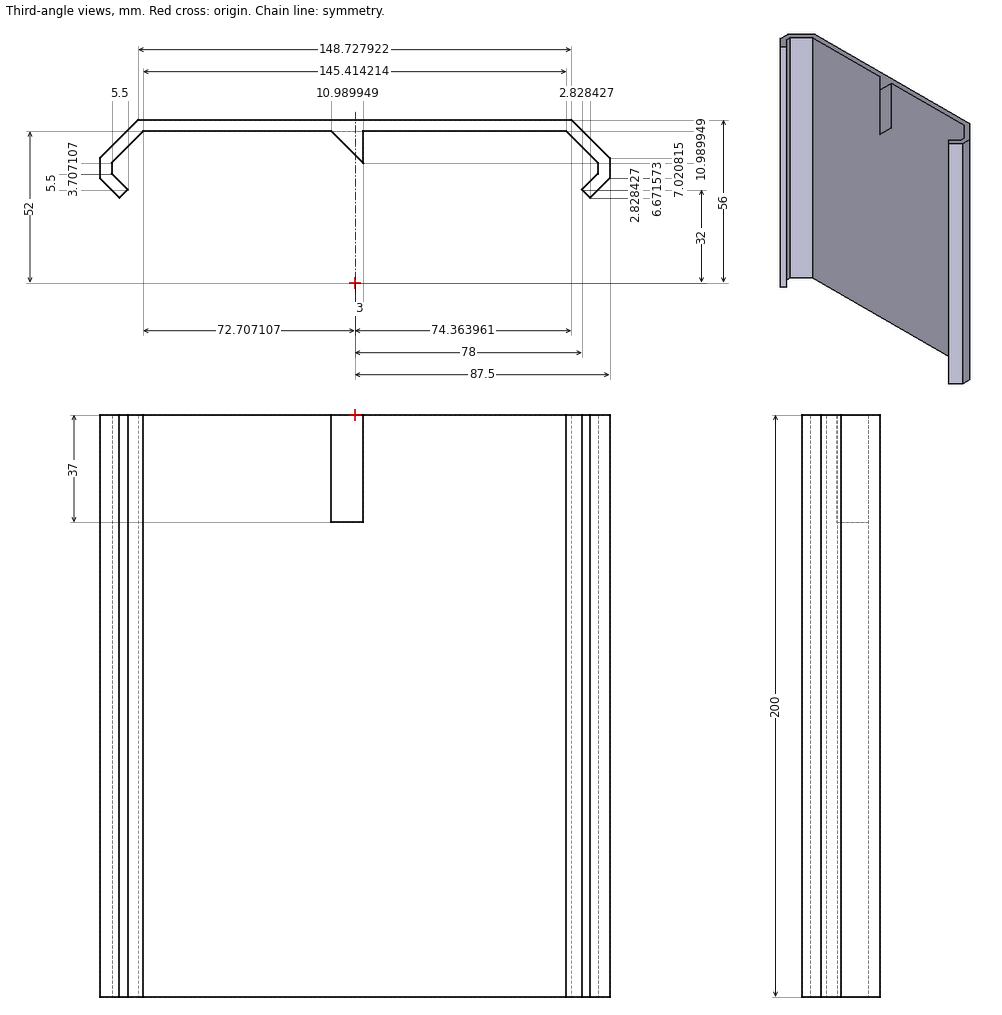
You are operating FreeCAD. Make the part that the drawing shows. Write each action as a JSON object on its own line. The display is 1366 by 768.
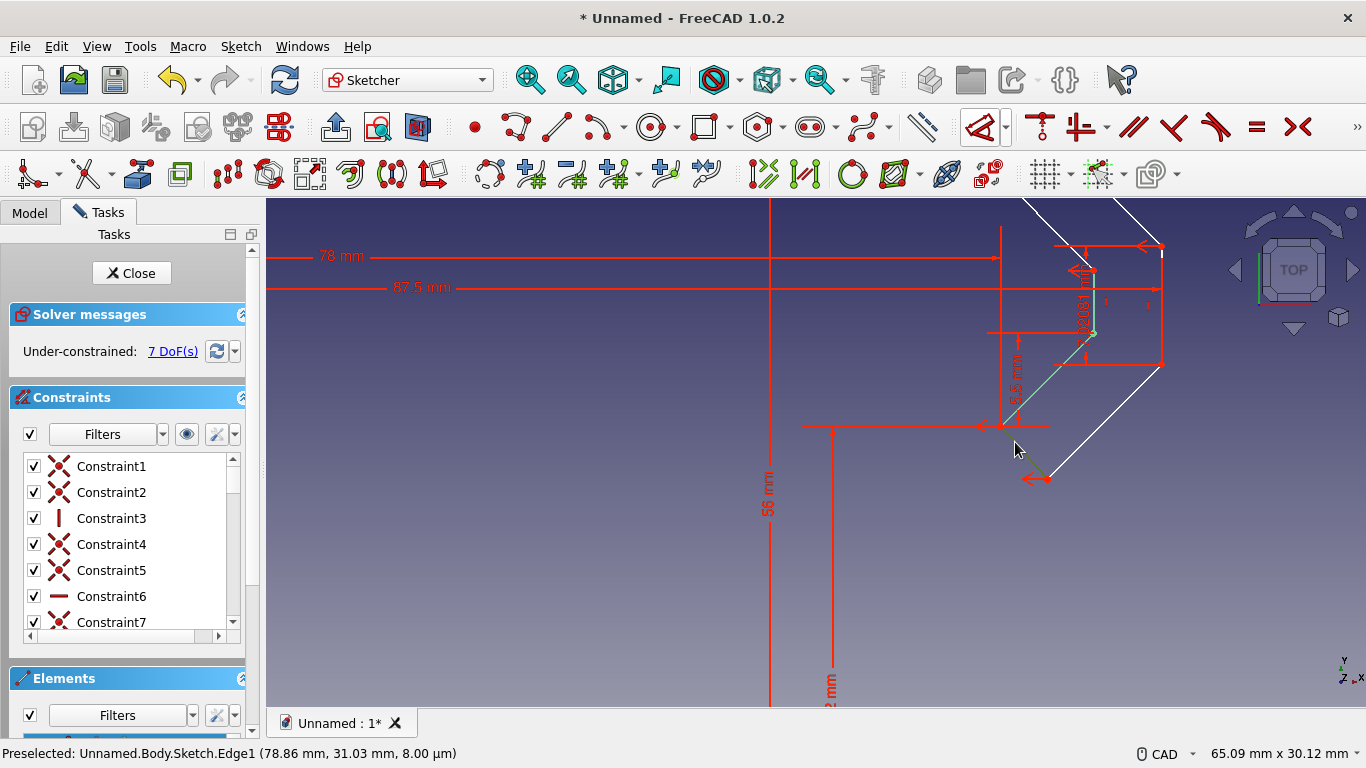
{"action": "left_click", "coordinate": [1006, 128]}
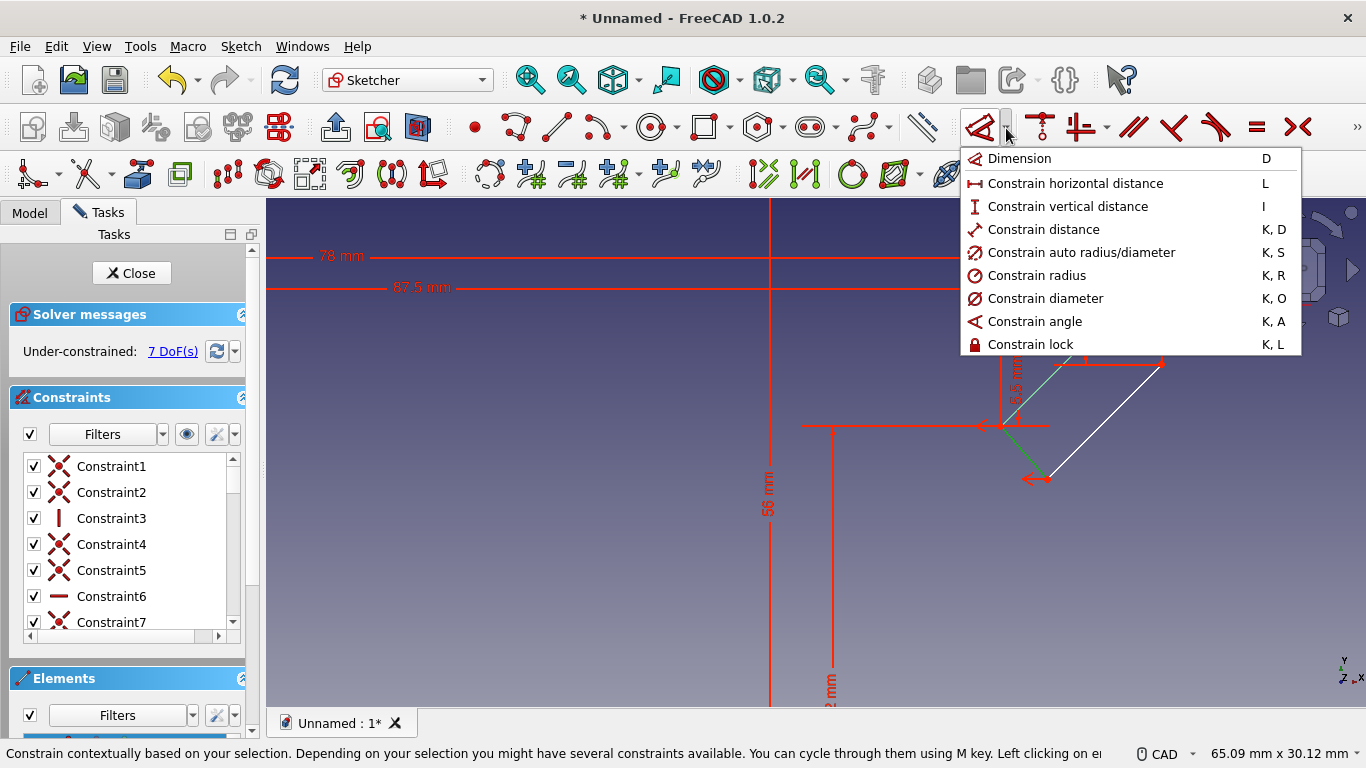
{"action": "left_click", "coordinate": [1131, 184]}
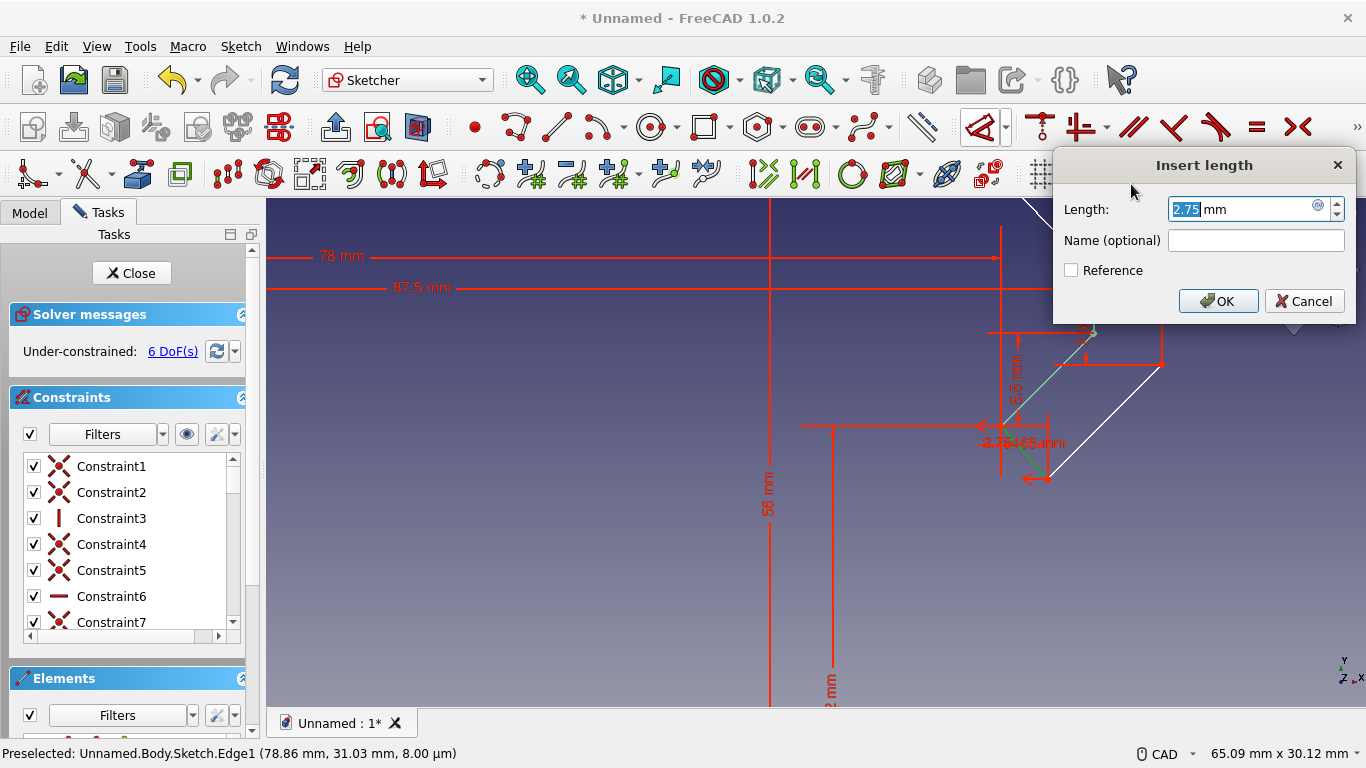
{"action": "type", "text": "2.828427"}
{"action": "key", "text": "Return"}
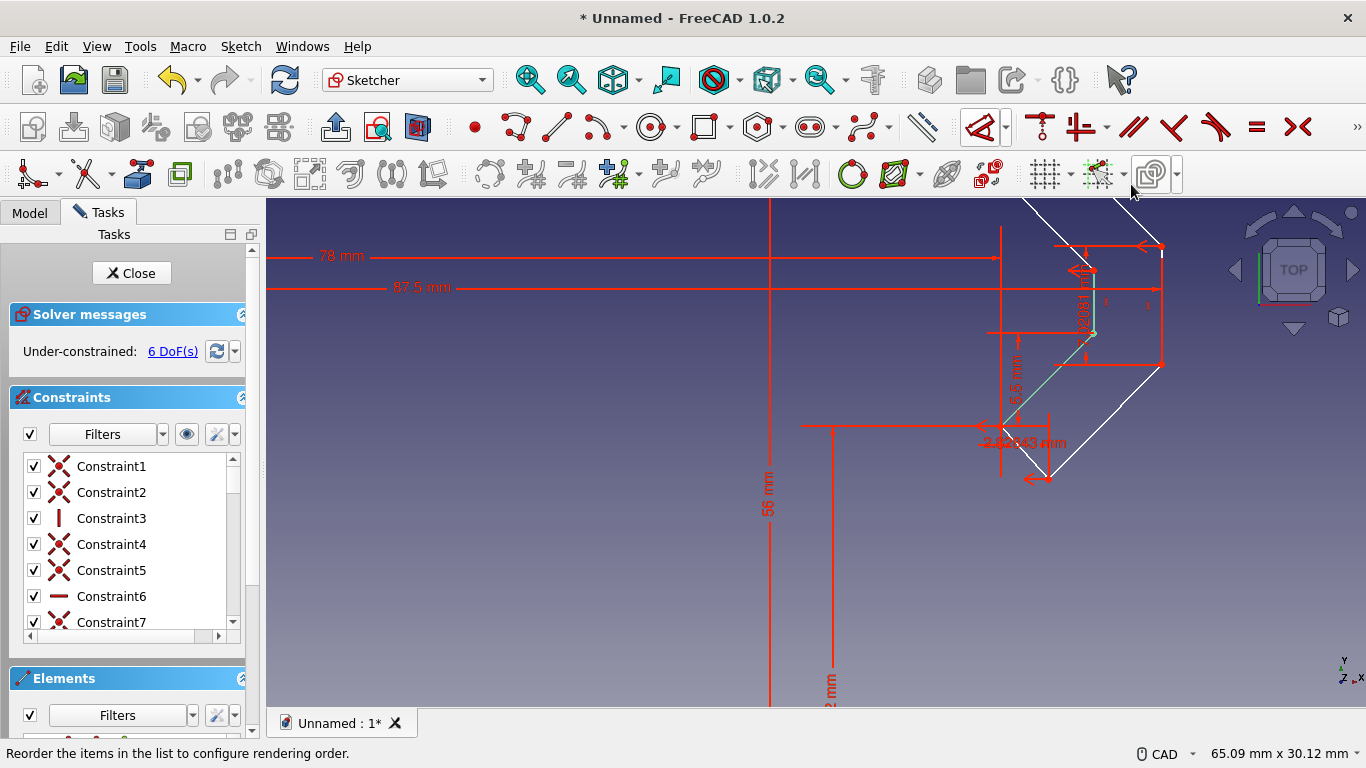
{"action": "left_click", "coordinate": [1034, 463]}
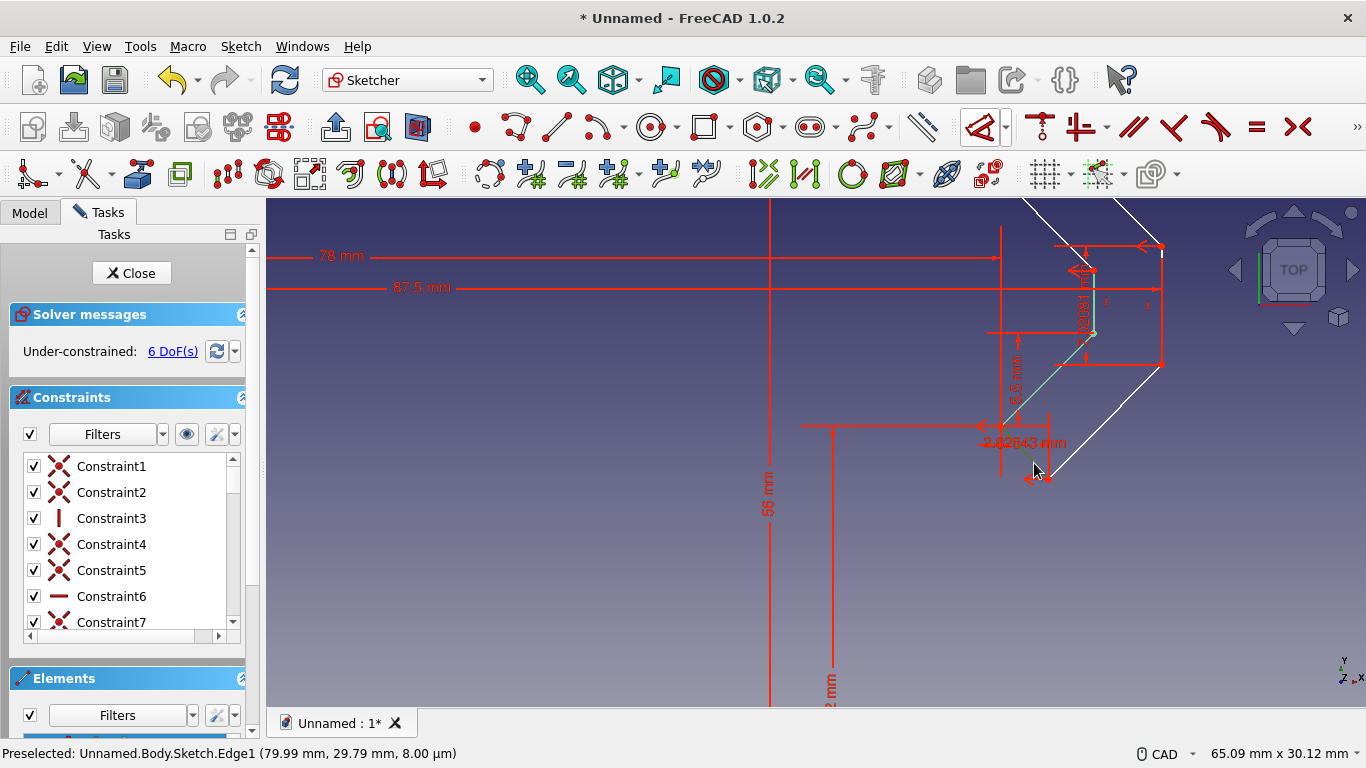
{"action": "left_click", "coordinate": [1006, 128]}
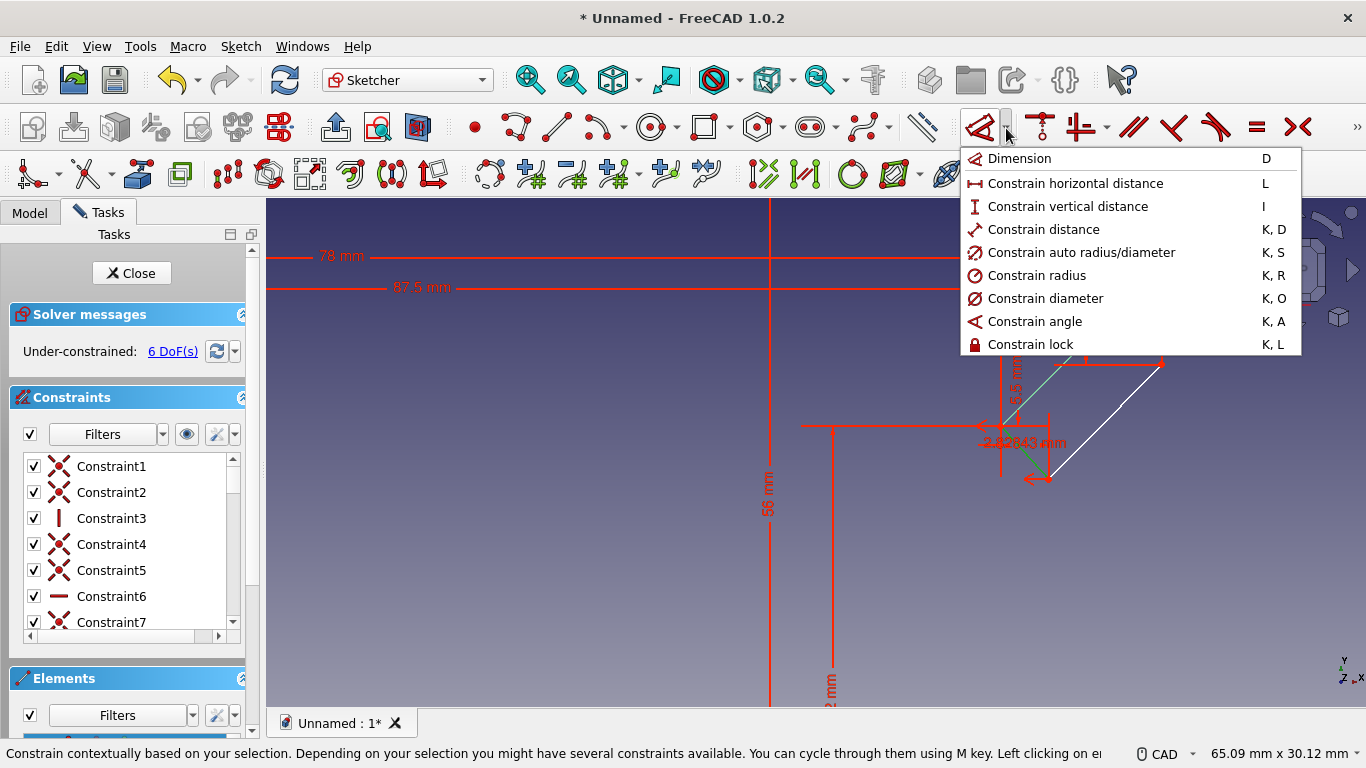
{"action": "left_click", "coordinate": [1131, 206]}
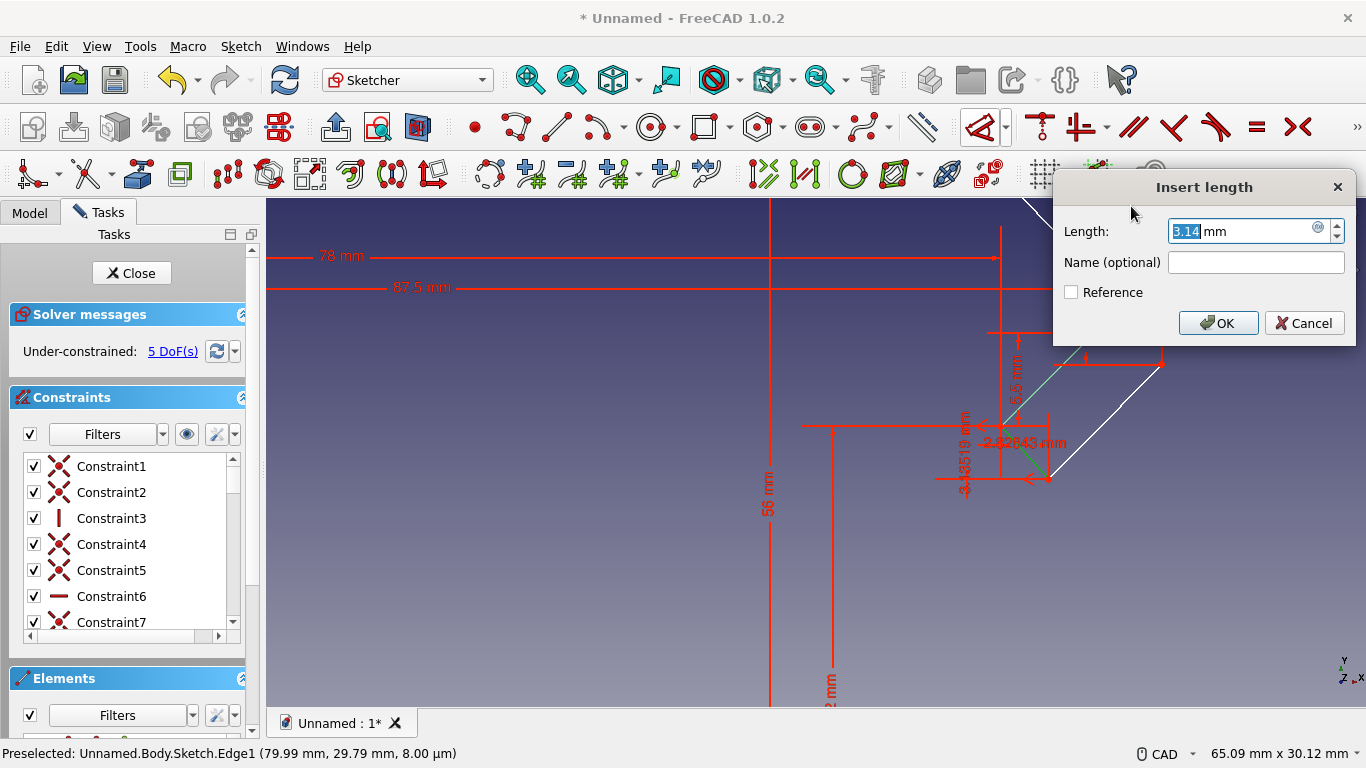
{"action": "type", "text": "2.828427"}
{"action": "key", "text": "Return"}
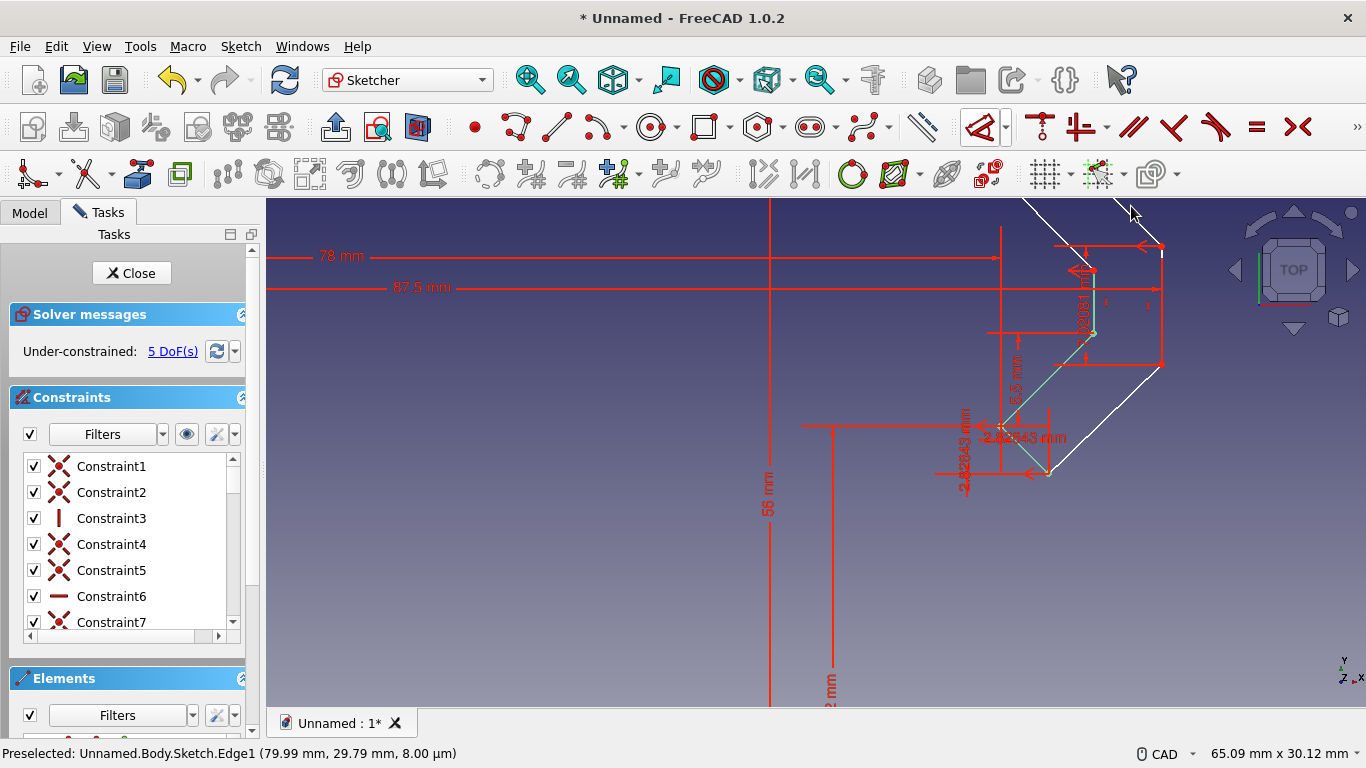
{"action": "left_click", "coordinate": [1083, 441]}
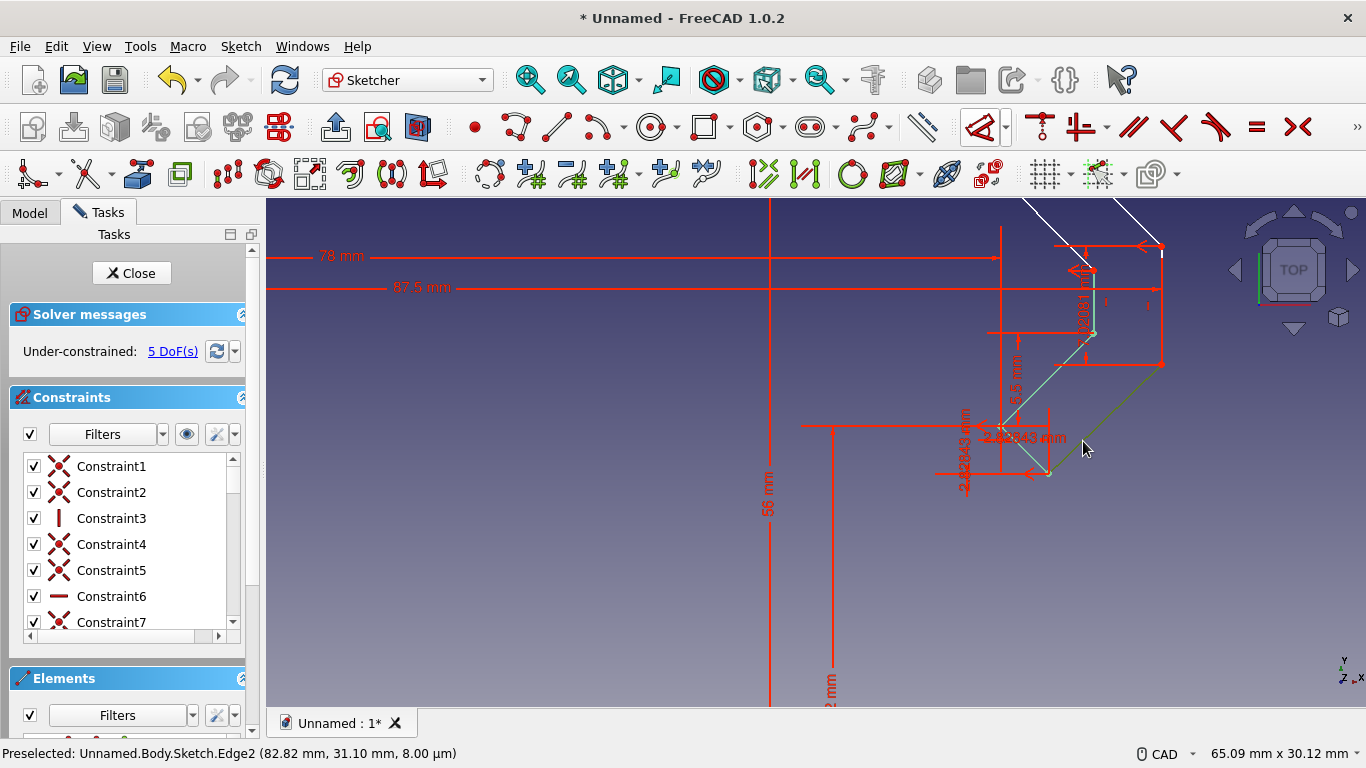
{"action": "left_click", "coordinate": [1006, 128]}